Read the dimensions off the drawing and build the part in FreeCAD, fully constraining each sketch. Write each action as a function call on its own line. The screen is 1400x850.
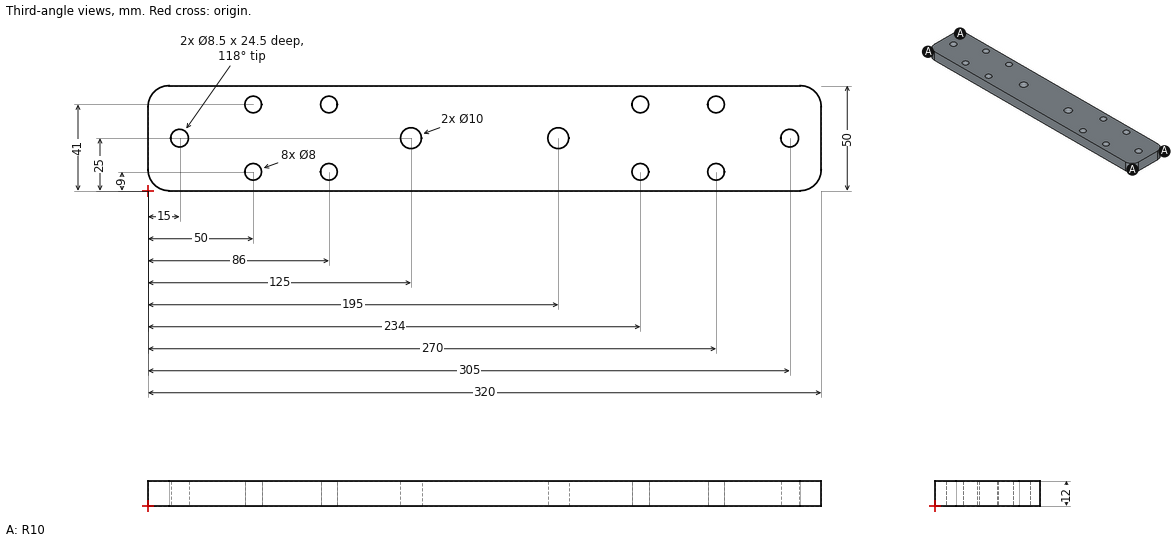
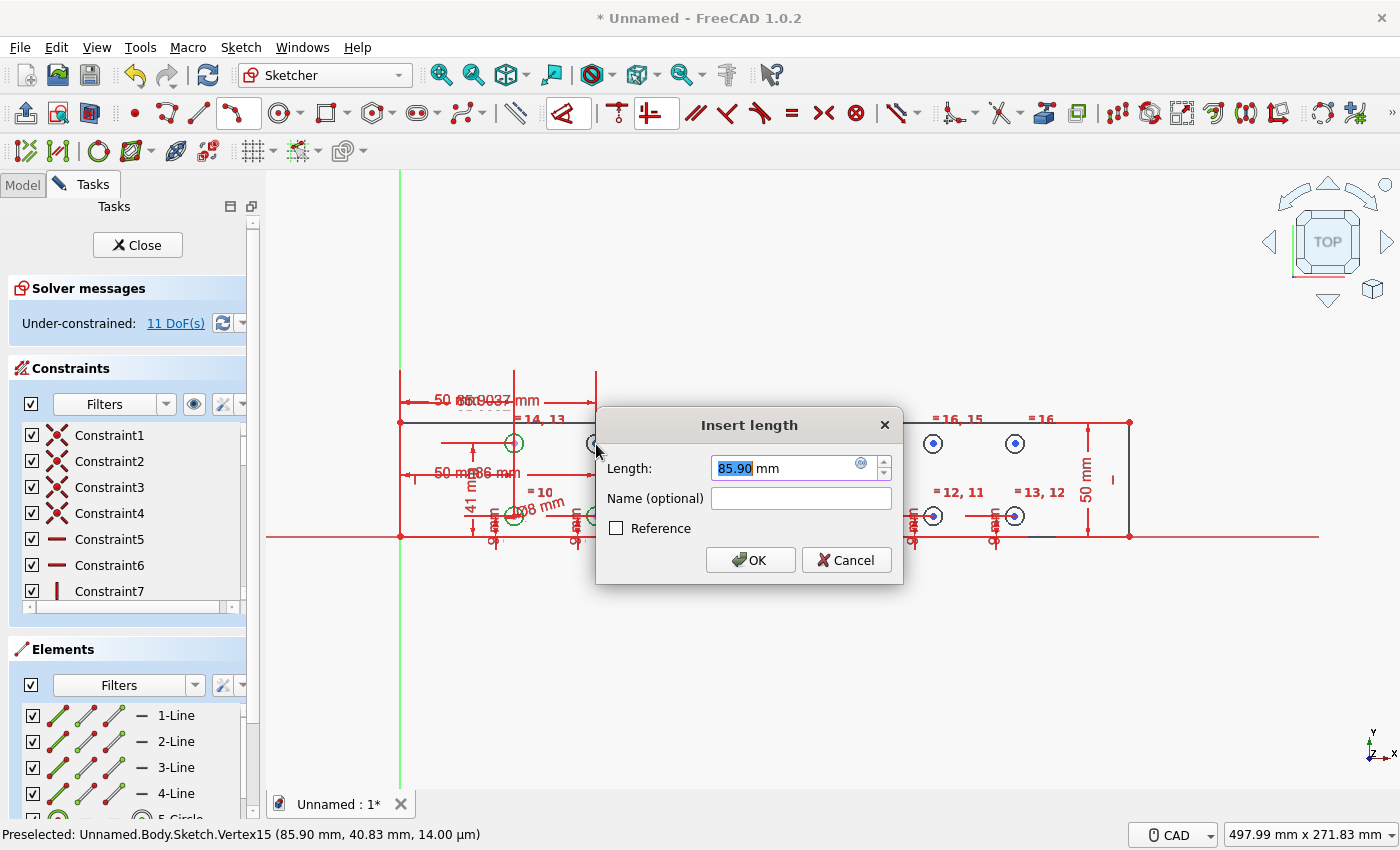
text(86)
key(Return)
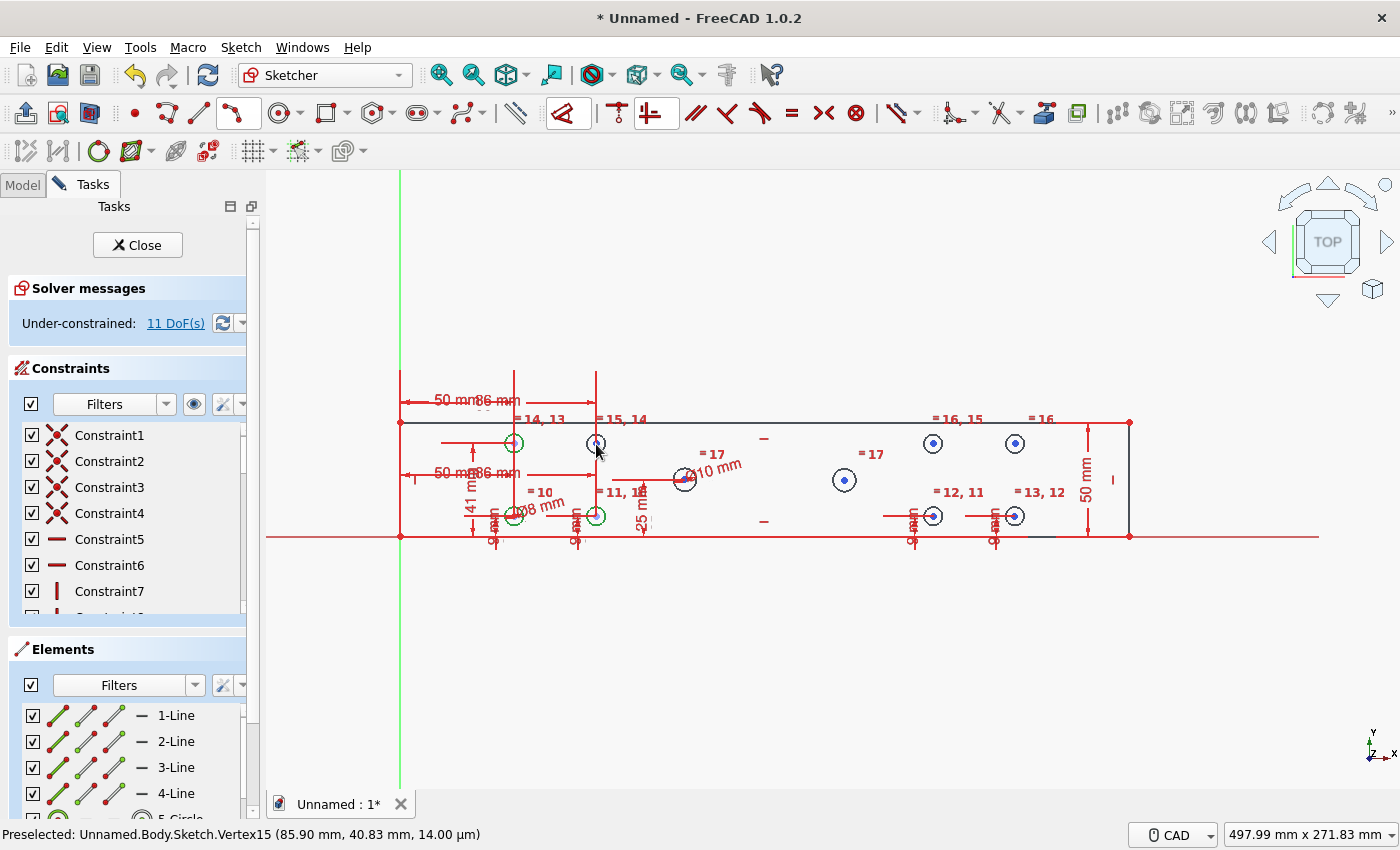
click(596, 444)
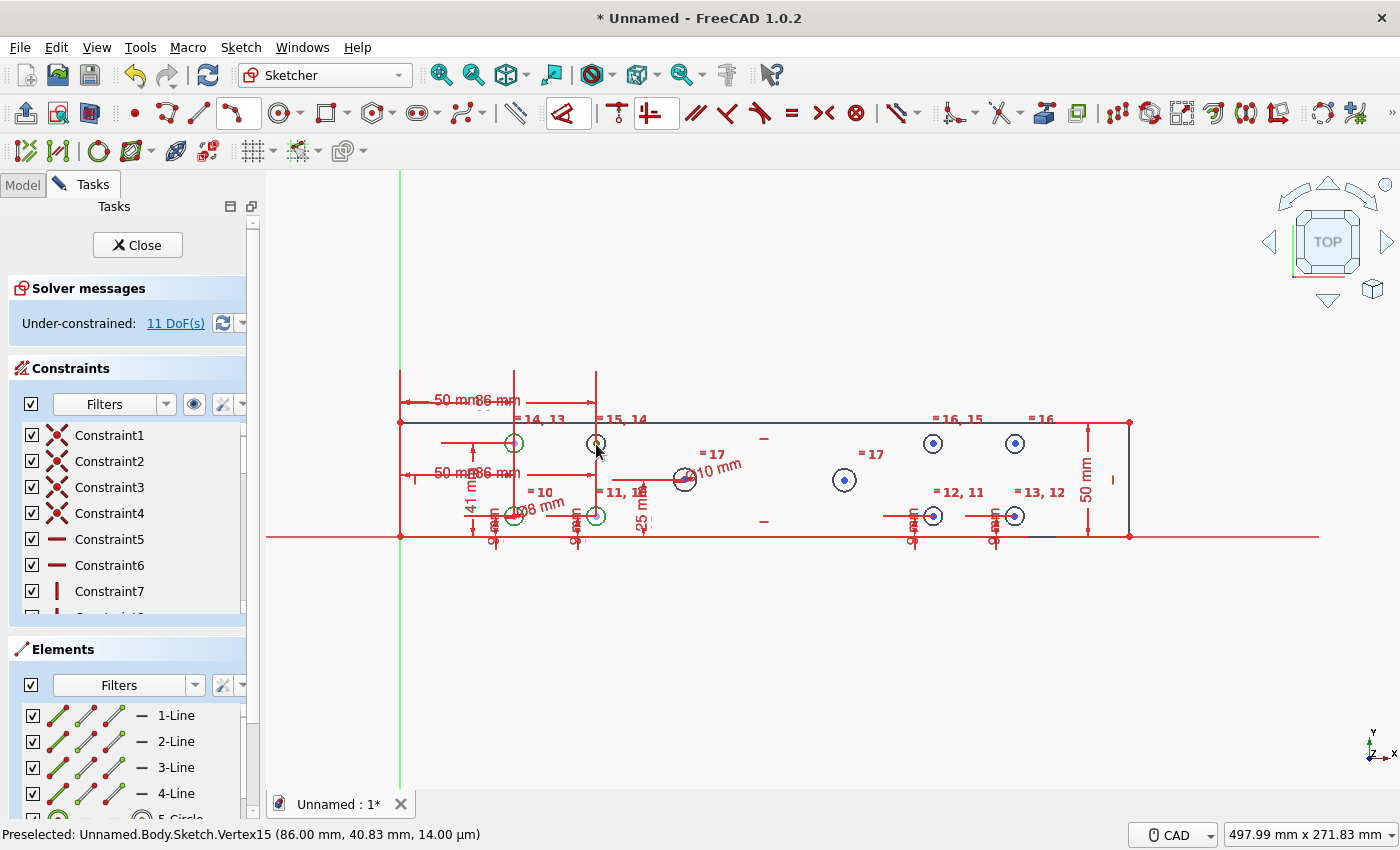
key(i)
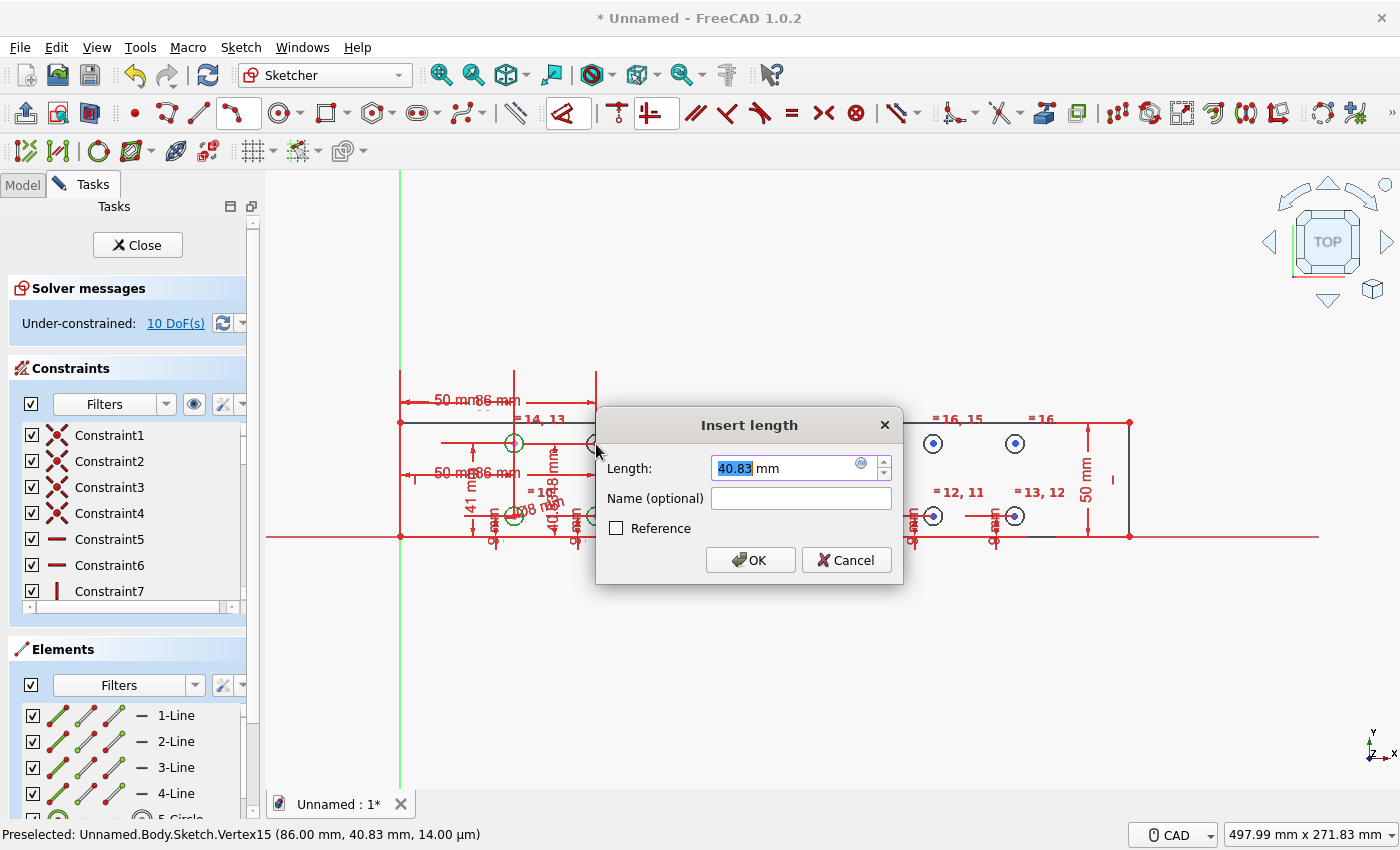
text(41)
key(Return)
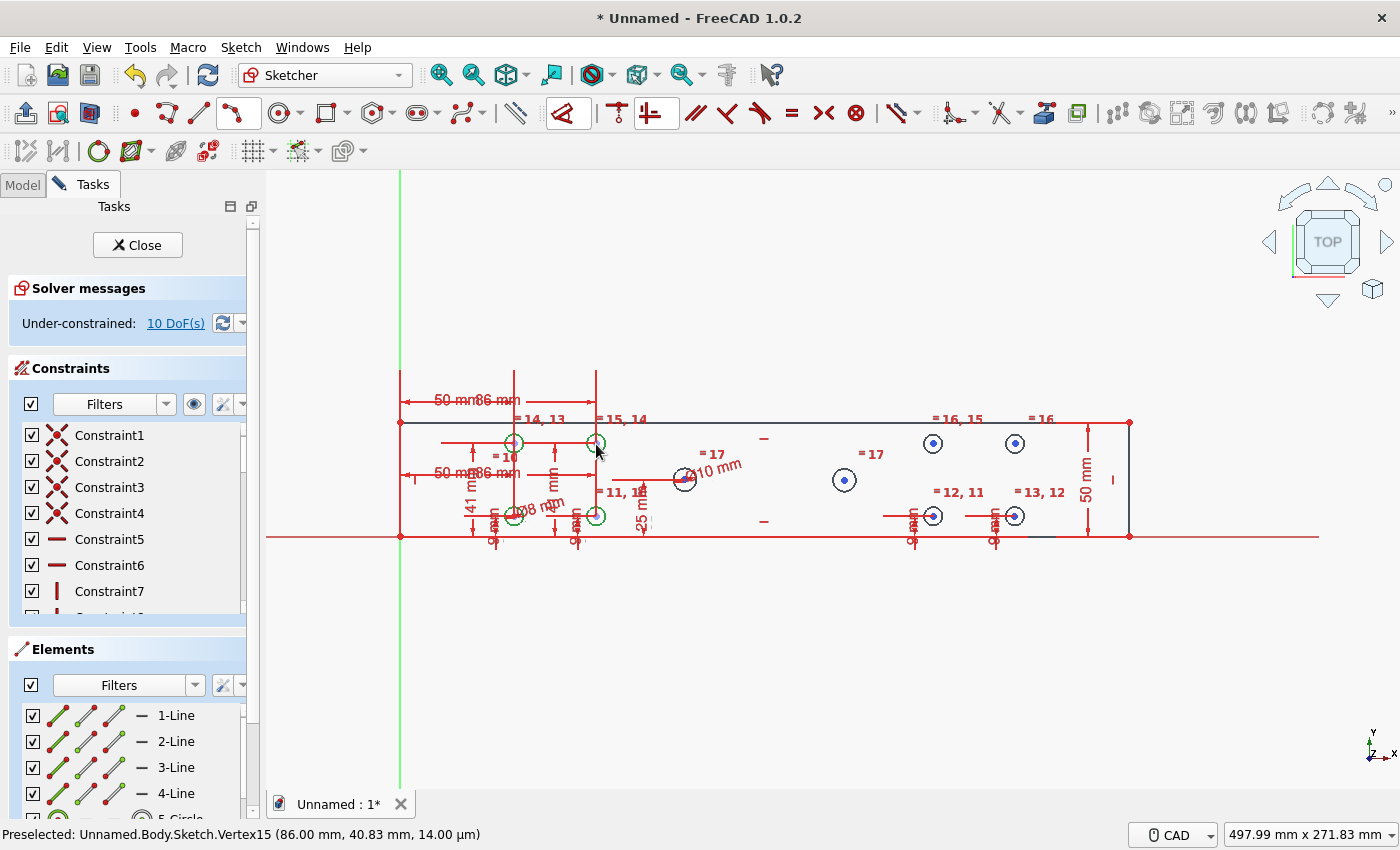
click(844, 480)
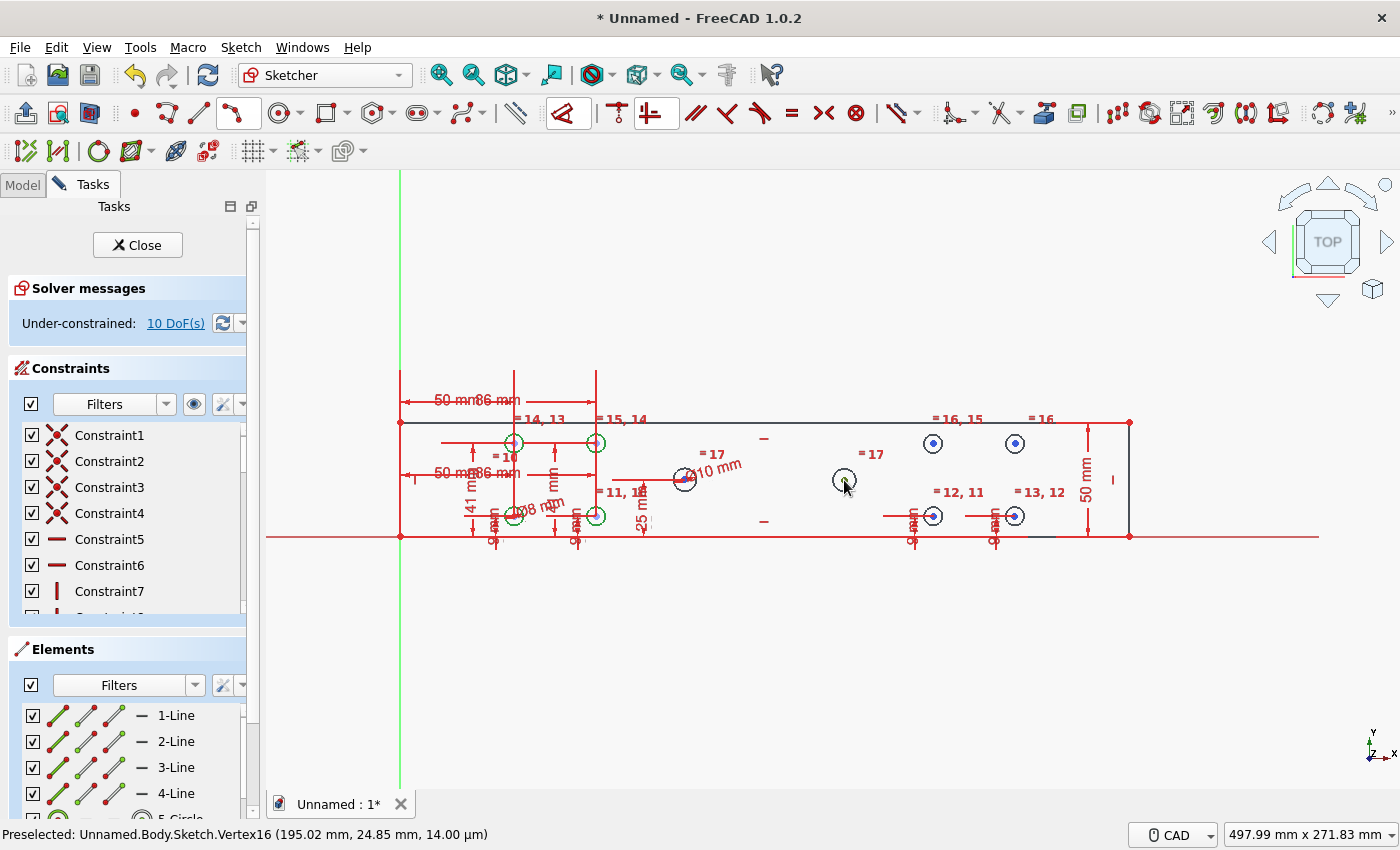
click(586, 114)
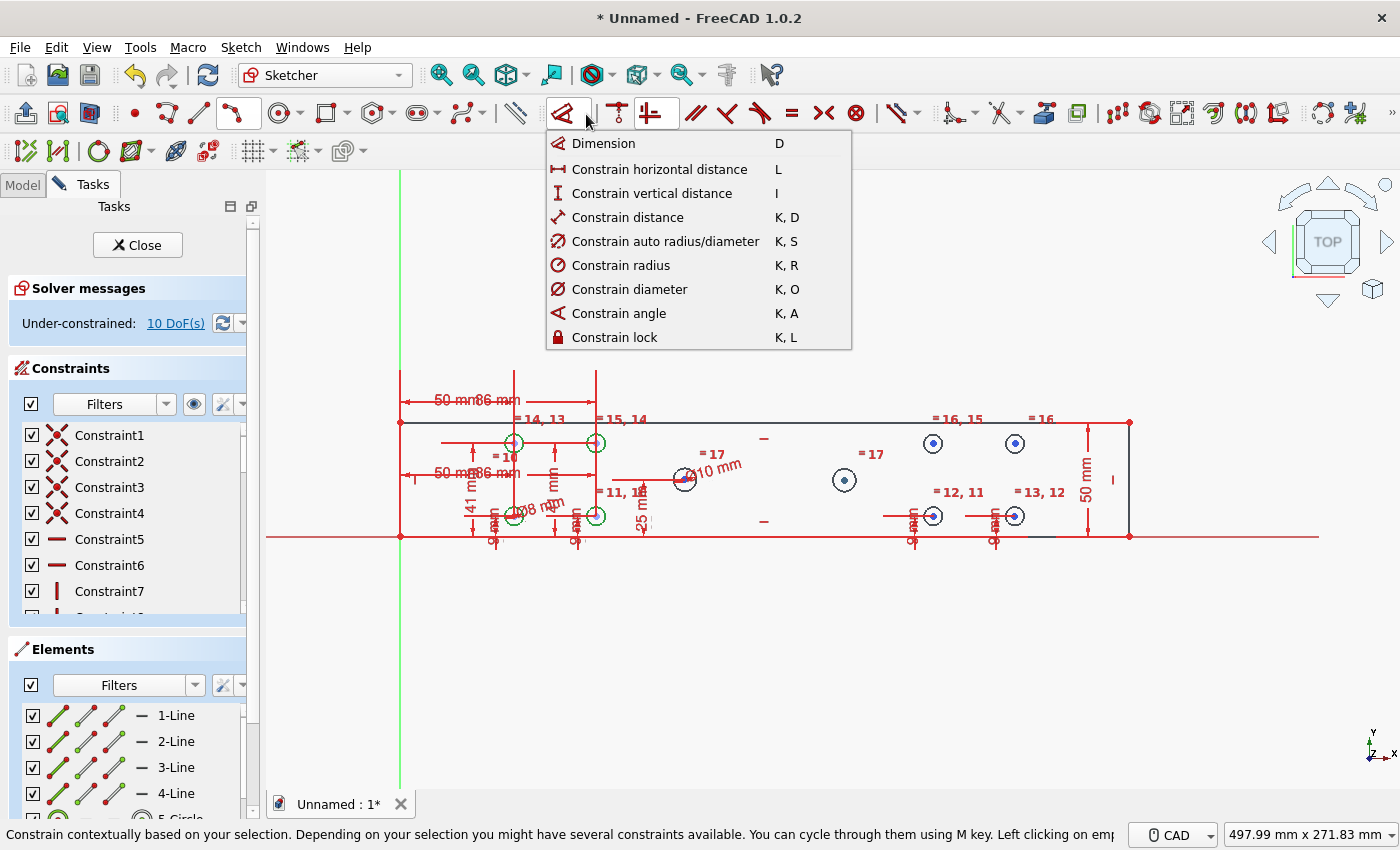
click(699, 193)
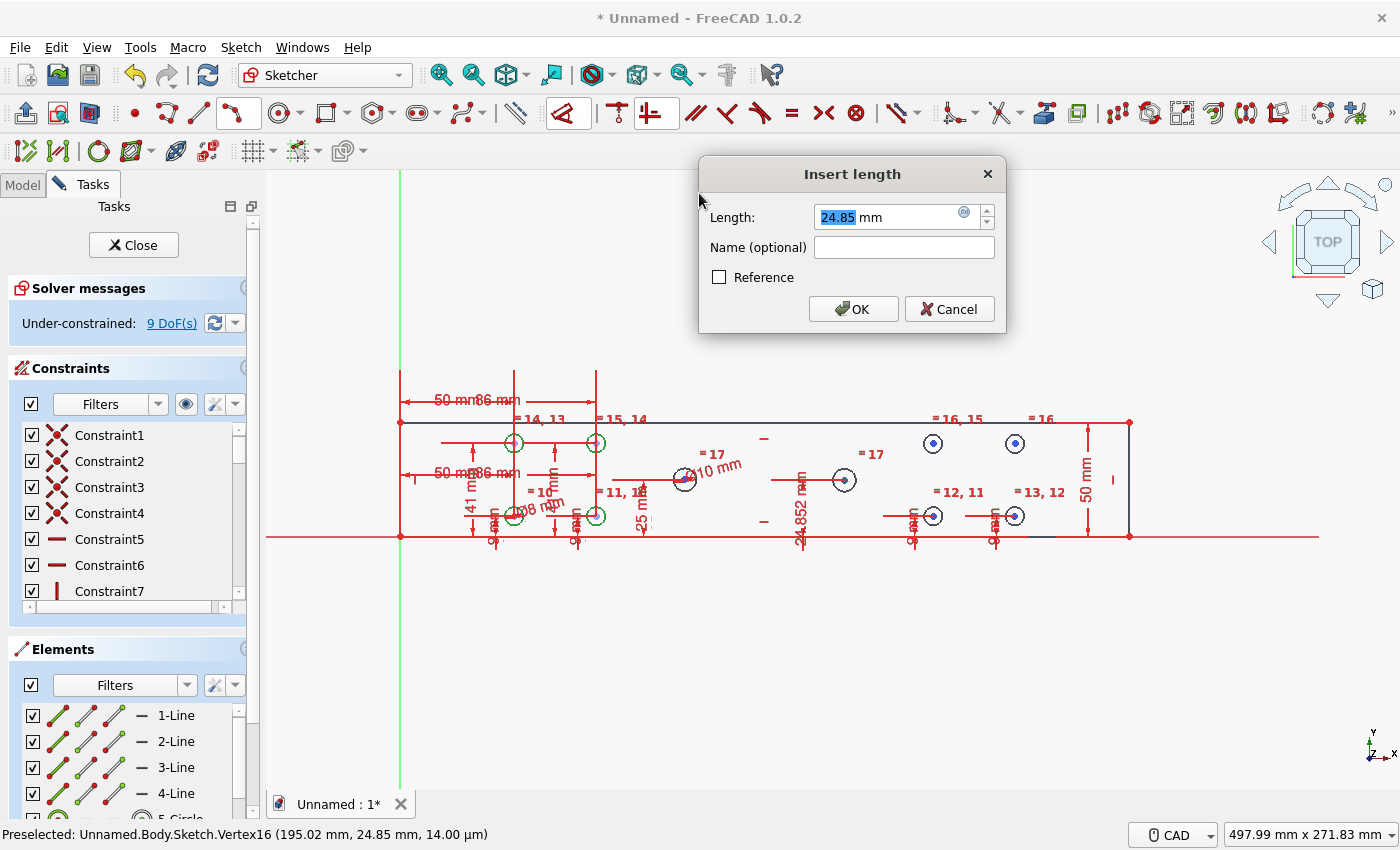
text(25)
key(Return)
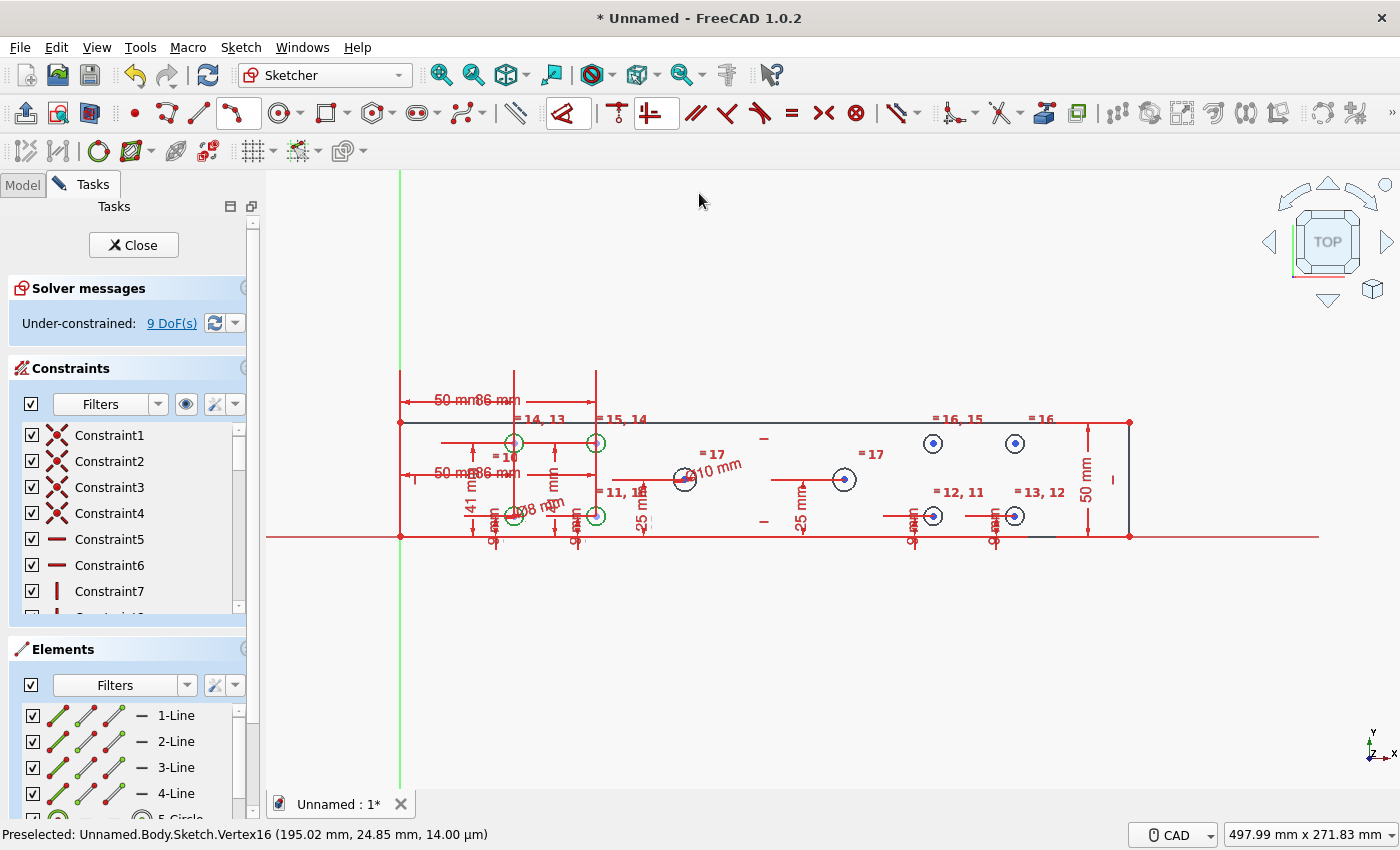
click(933, 444)